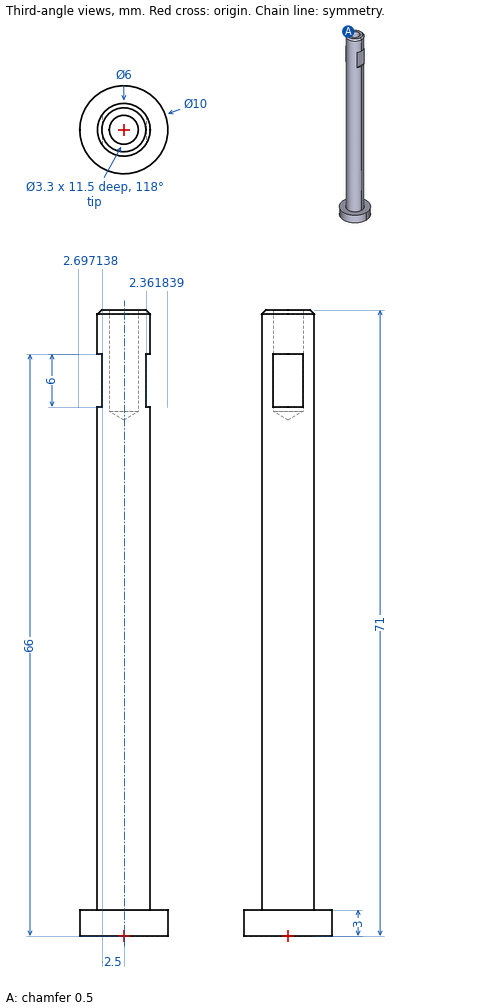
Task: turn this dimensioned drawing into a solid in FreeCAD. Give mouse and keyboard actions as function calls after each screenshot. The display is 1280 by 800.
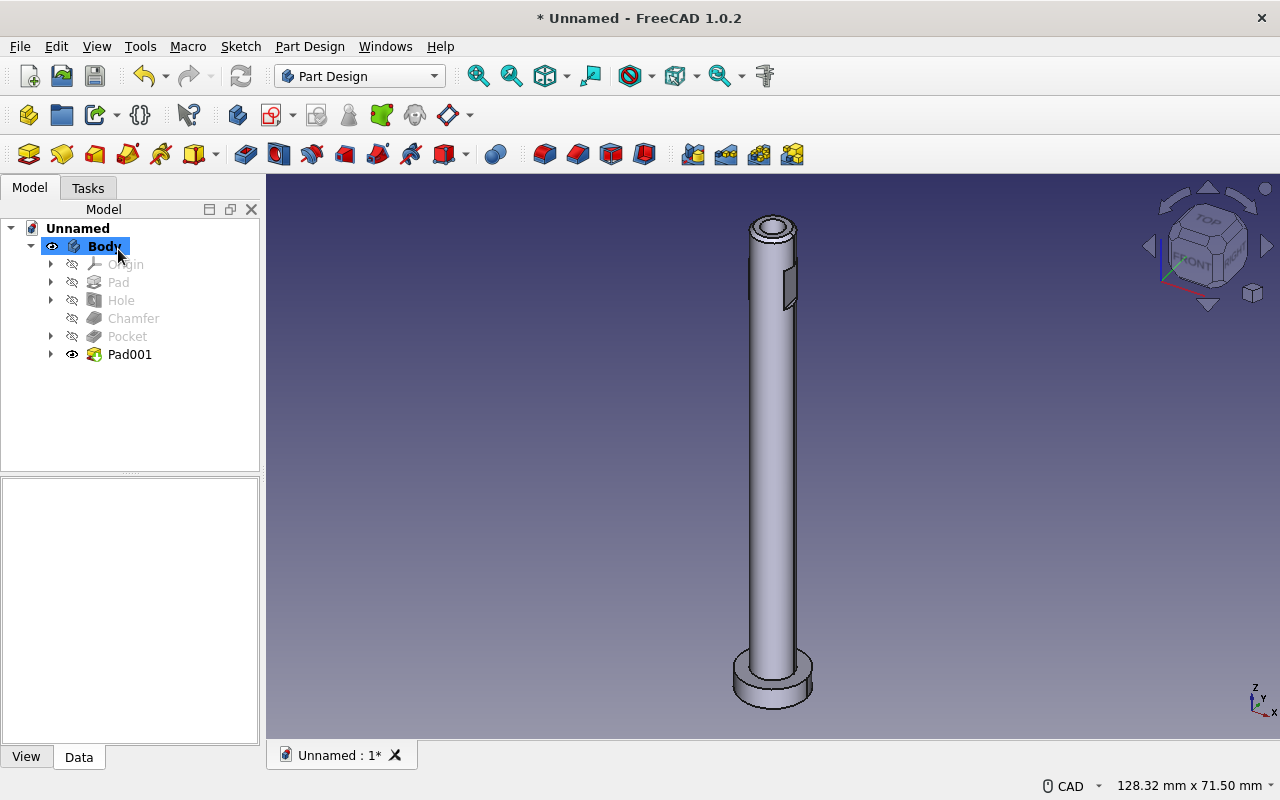
key(0)